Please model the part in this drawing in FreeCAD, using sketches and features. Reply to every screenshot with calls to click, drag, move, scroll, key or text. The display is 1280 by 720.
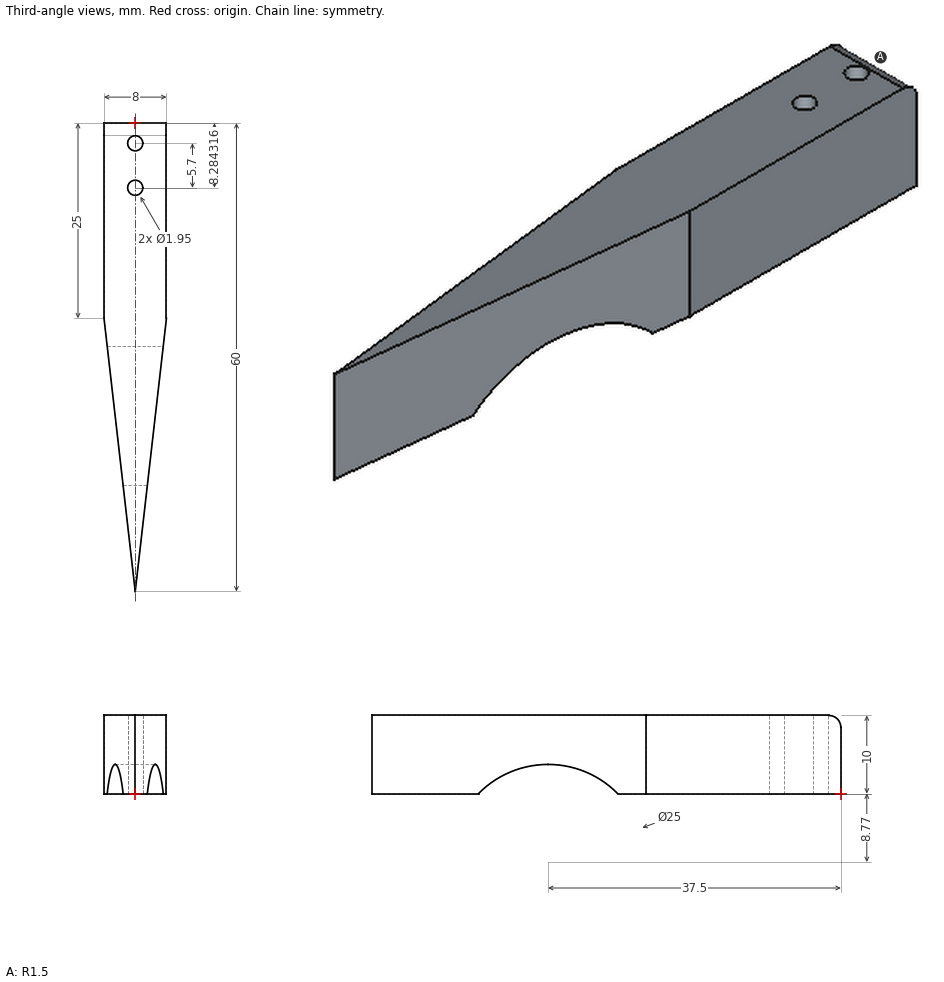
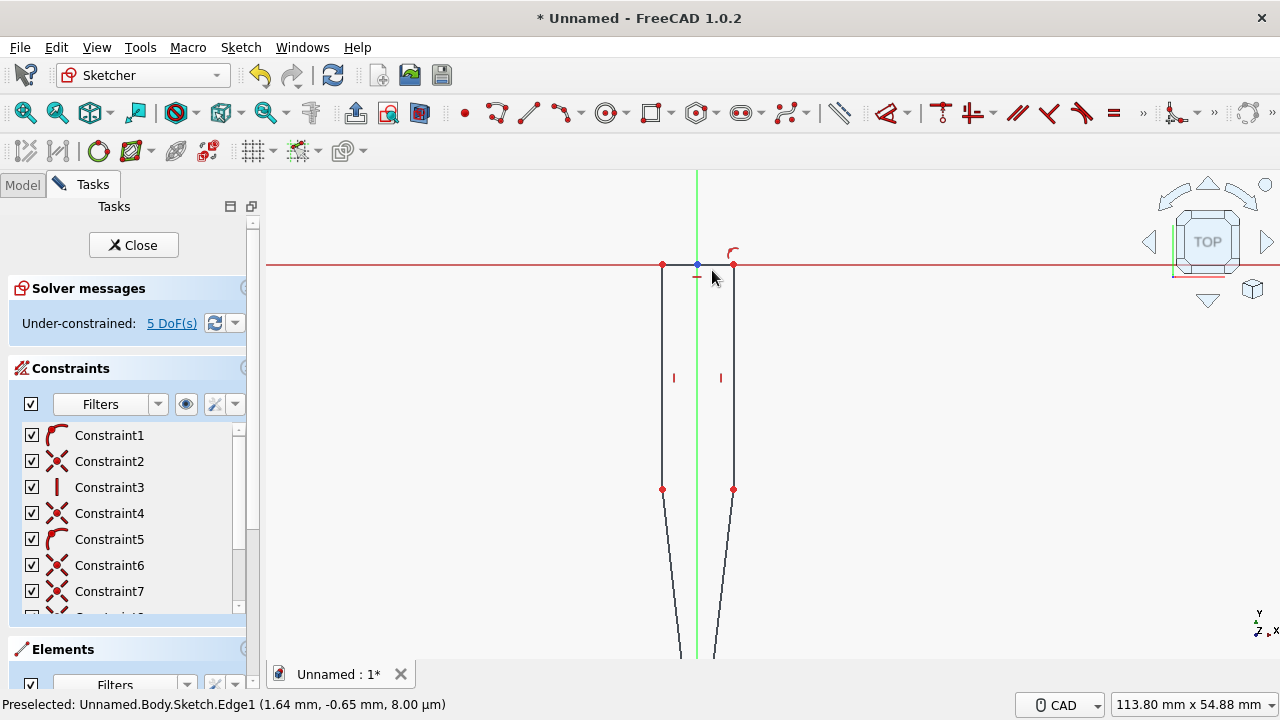
click(662, 489)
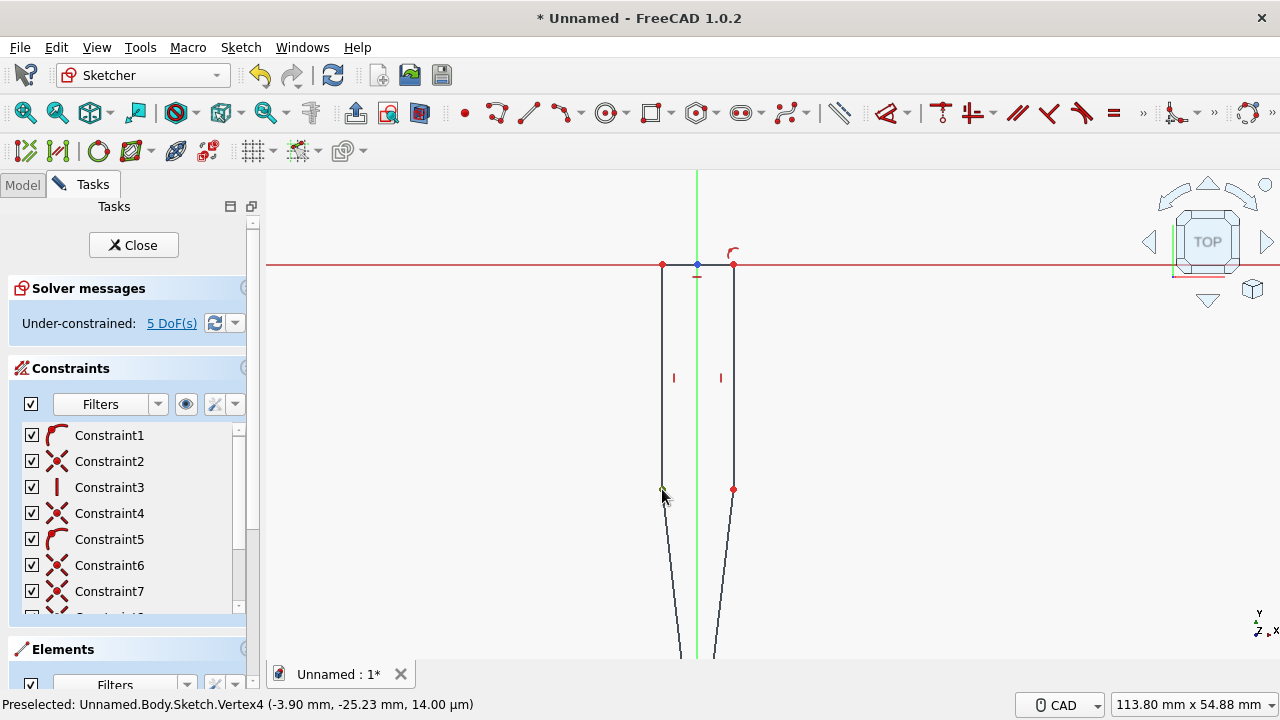
click(734, 489)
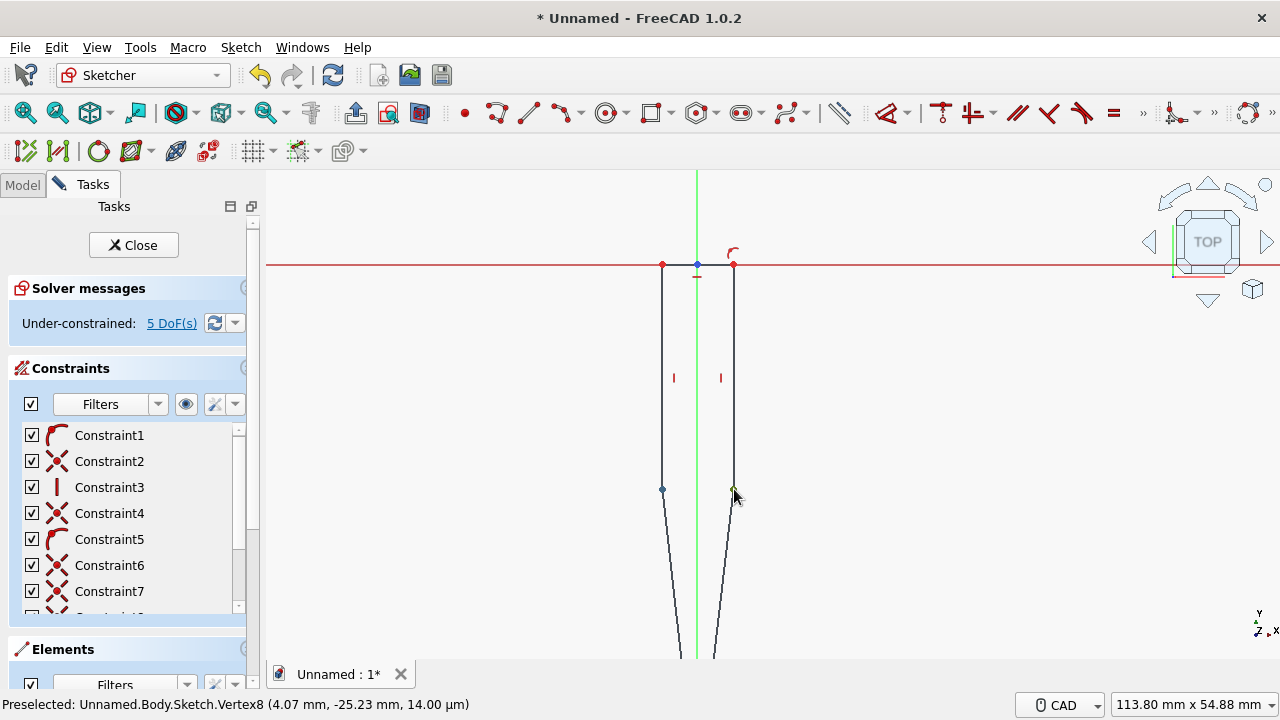
click(697, 507)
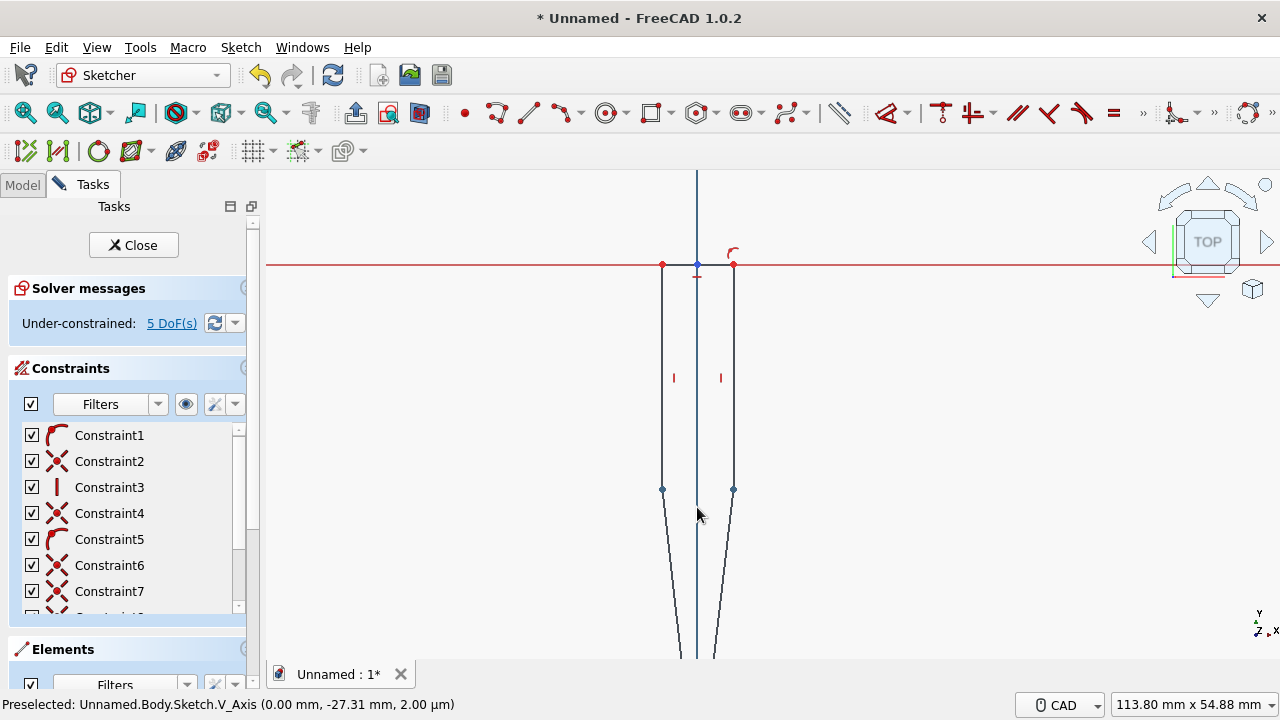
key(s)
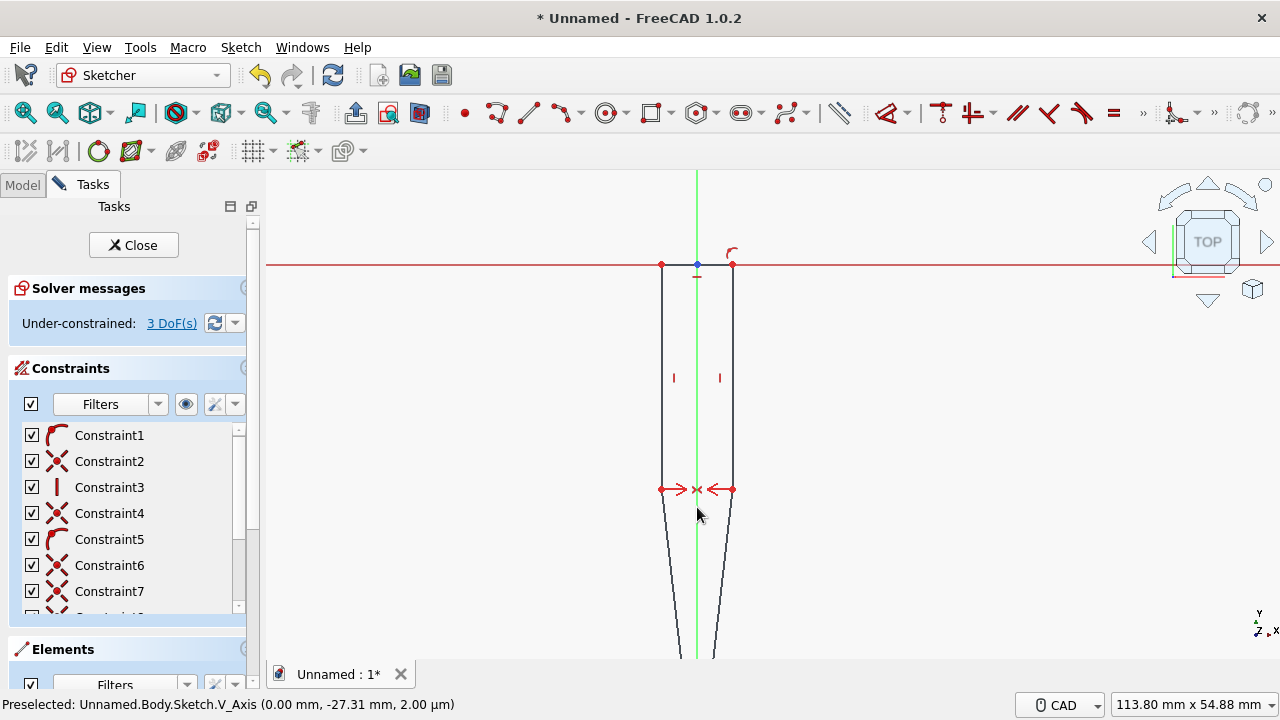
click(886, 114)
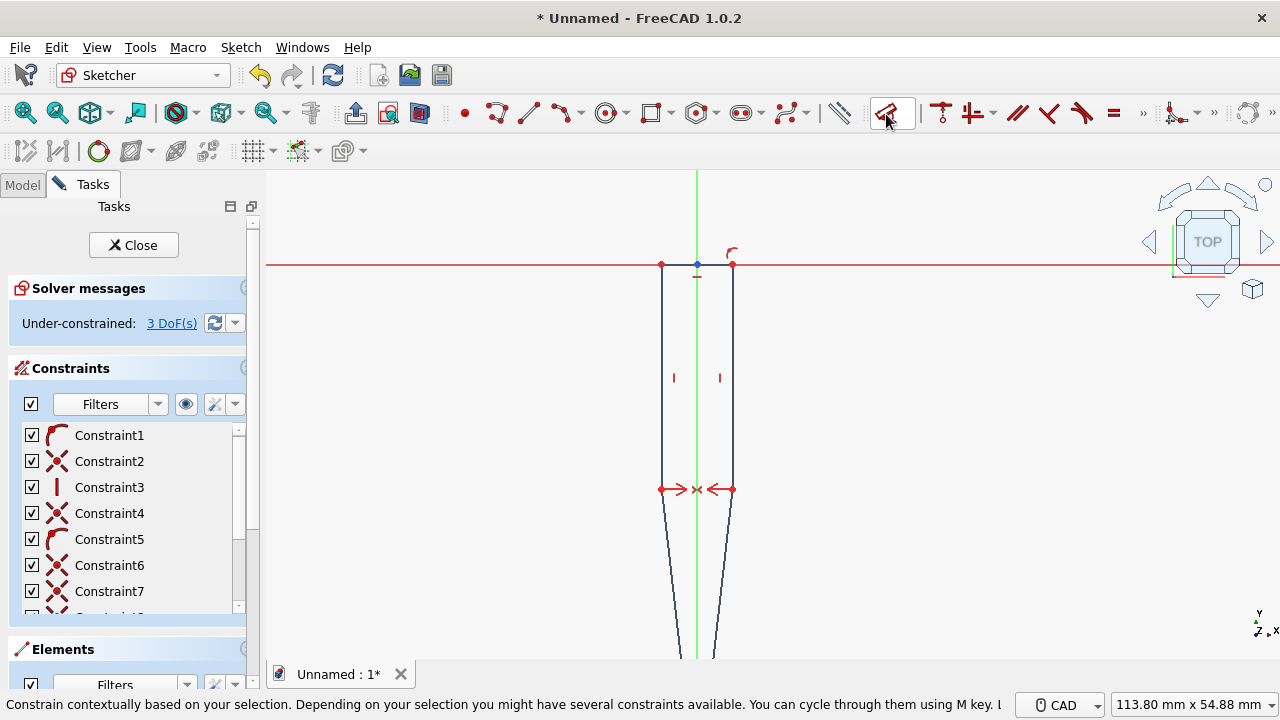
click(711, 265)
click(681, 231)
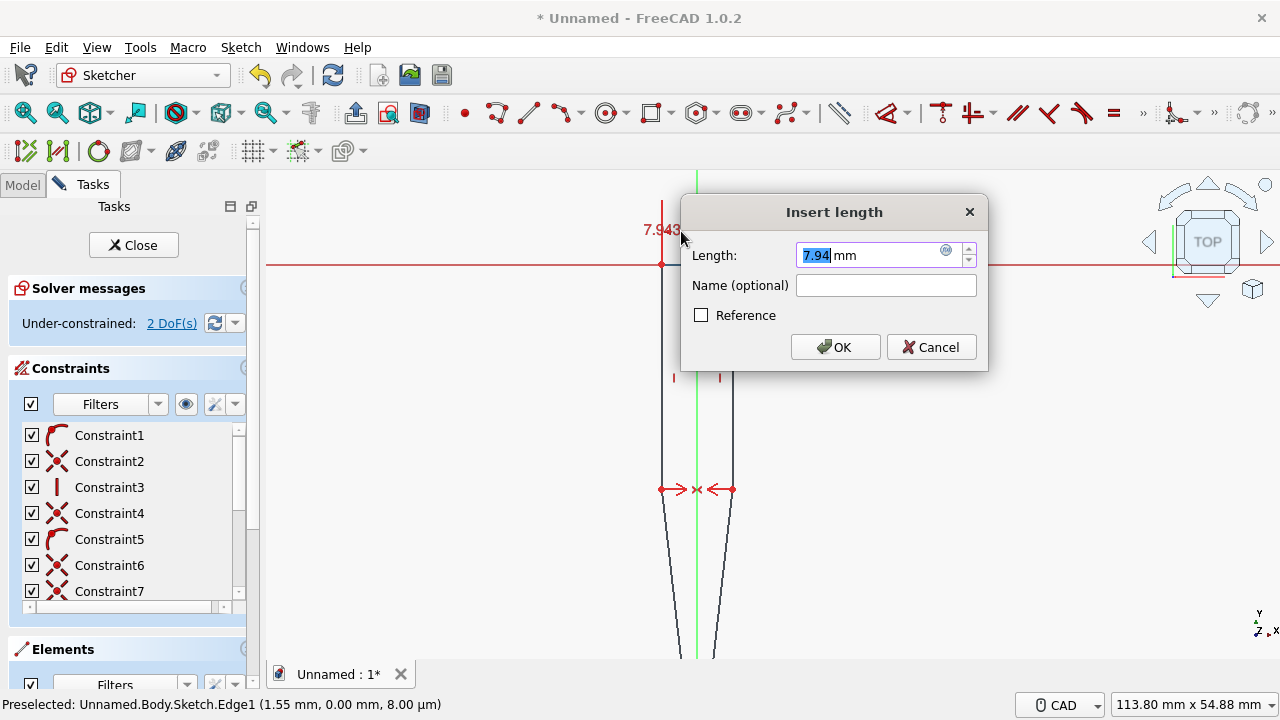
text(8)
key(Return)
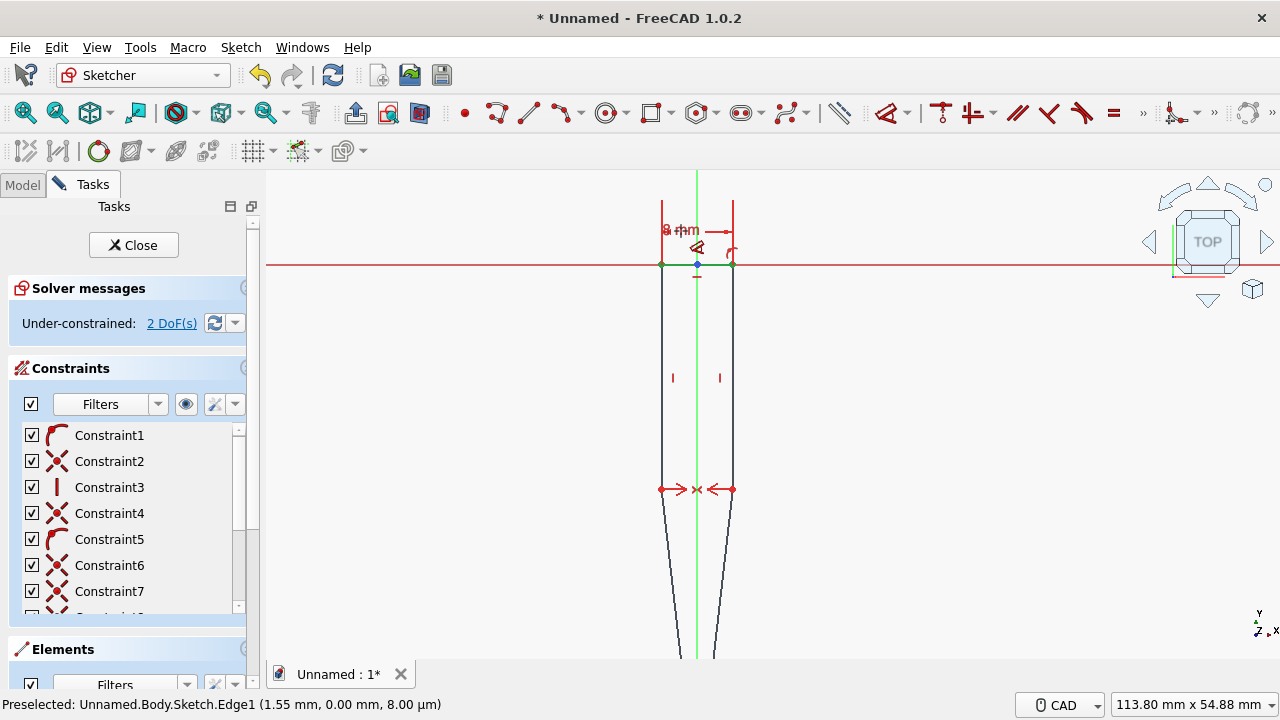
click(662, 332)
click(628, 377)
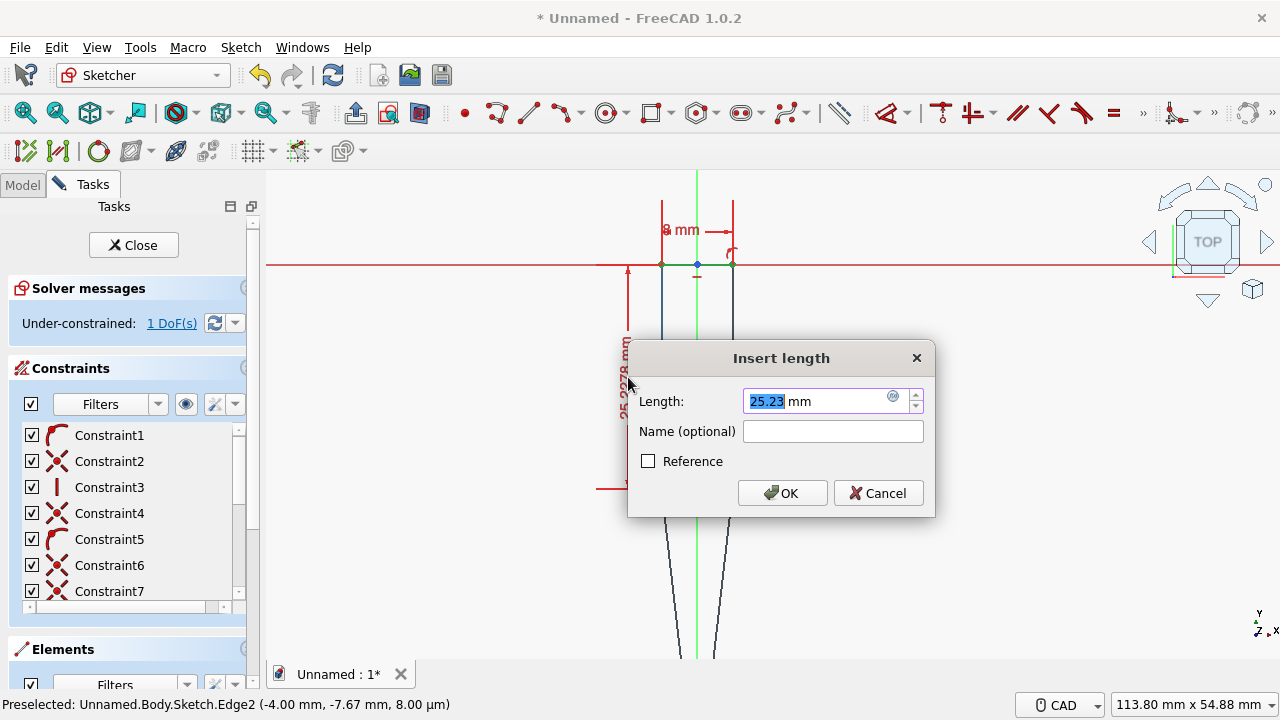
text(25)
key(Return)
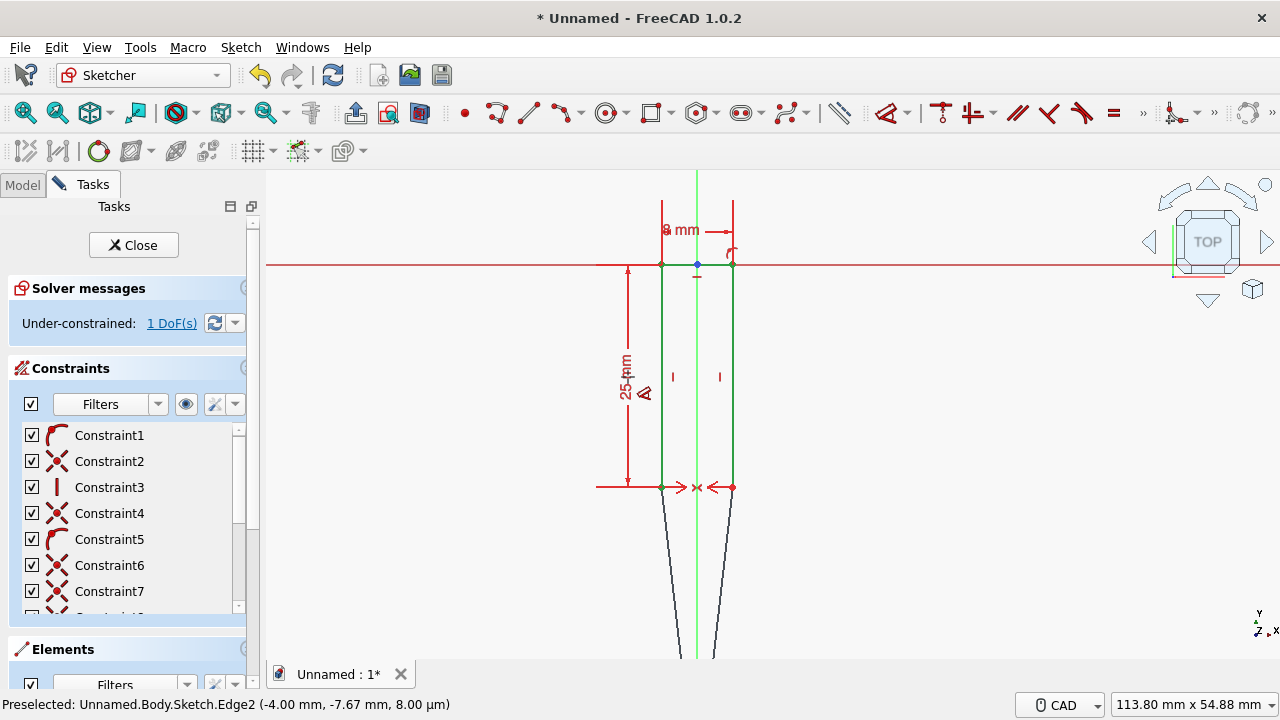
scroll(713, 272, down, 3)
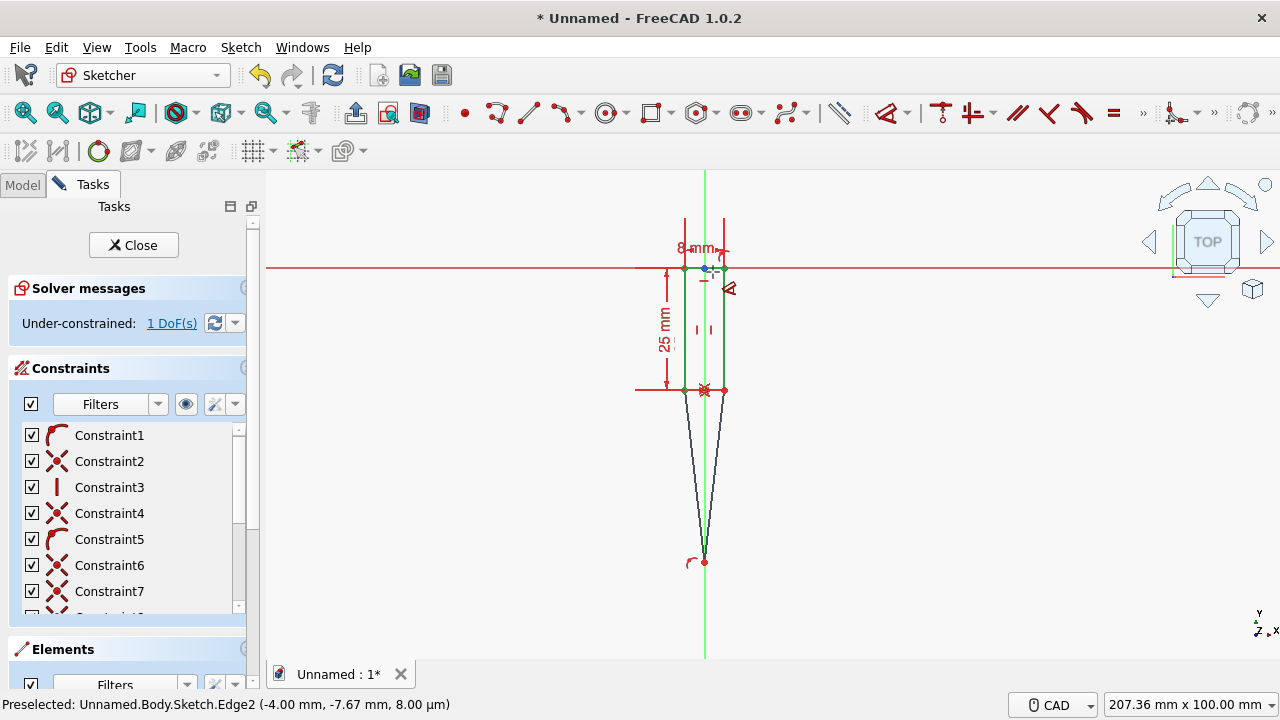
click(705, 562)
click(739, 415)